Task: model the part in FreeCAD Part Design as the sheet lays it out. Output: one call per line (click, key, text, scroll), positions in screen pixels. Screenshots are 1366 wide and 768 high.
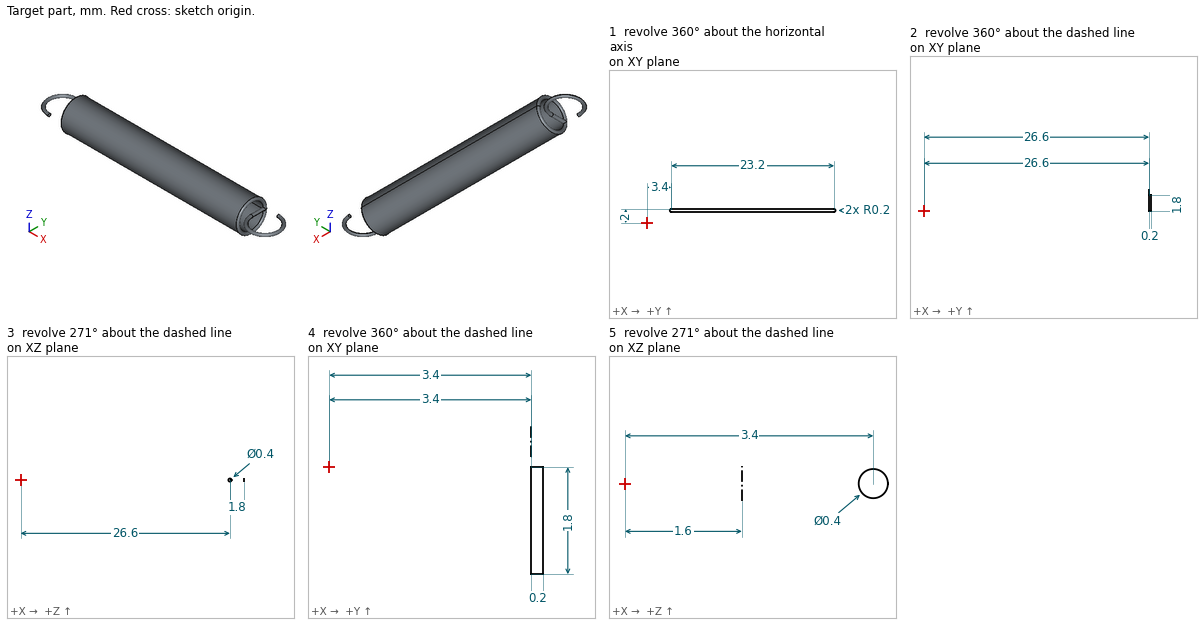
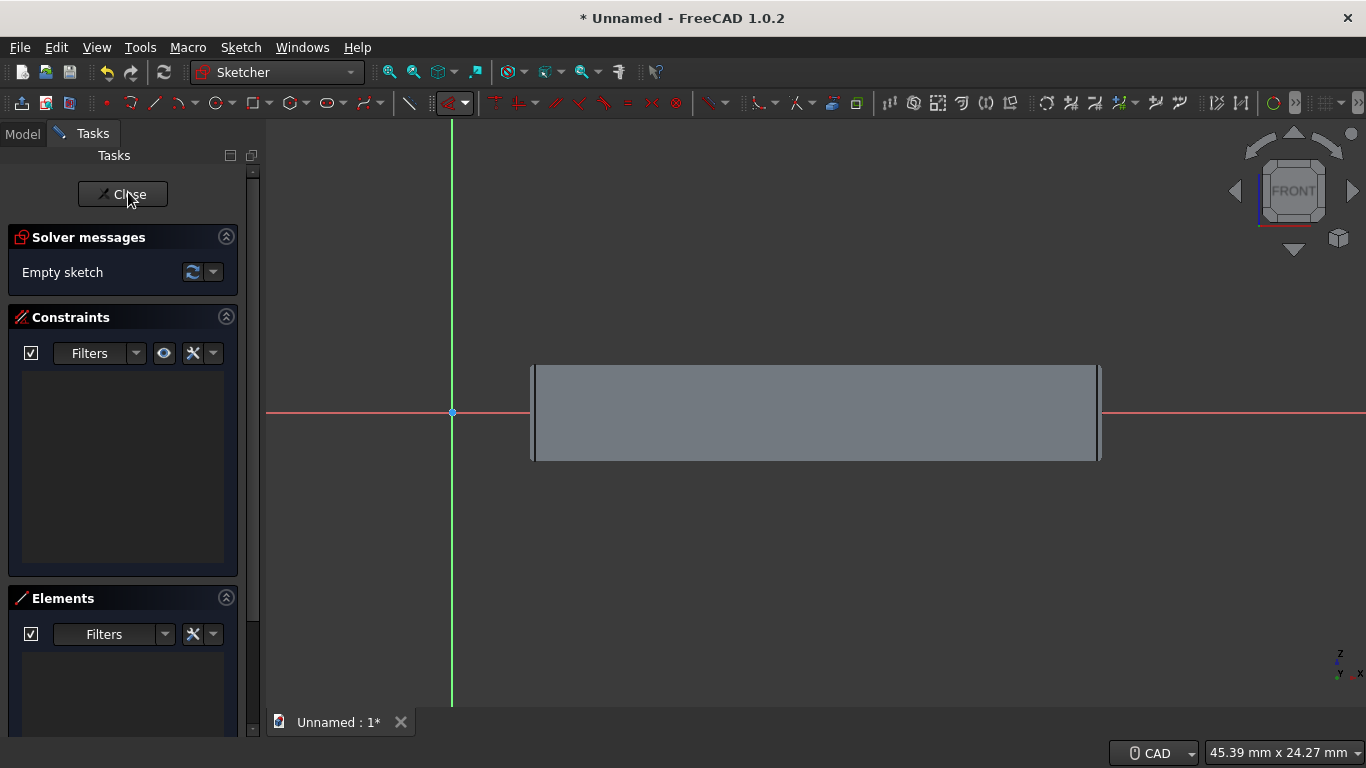
click(70, 104)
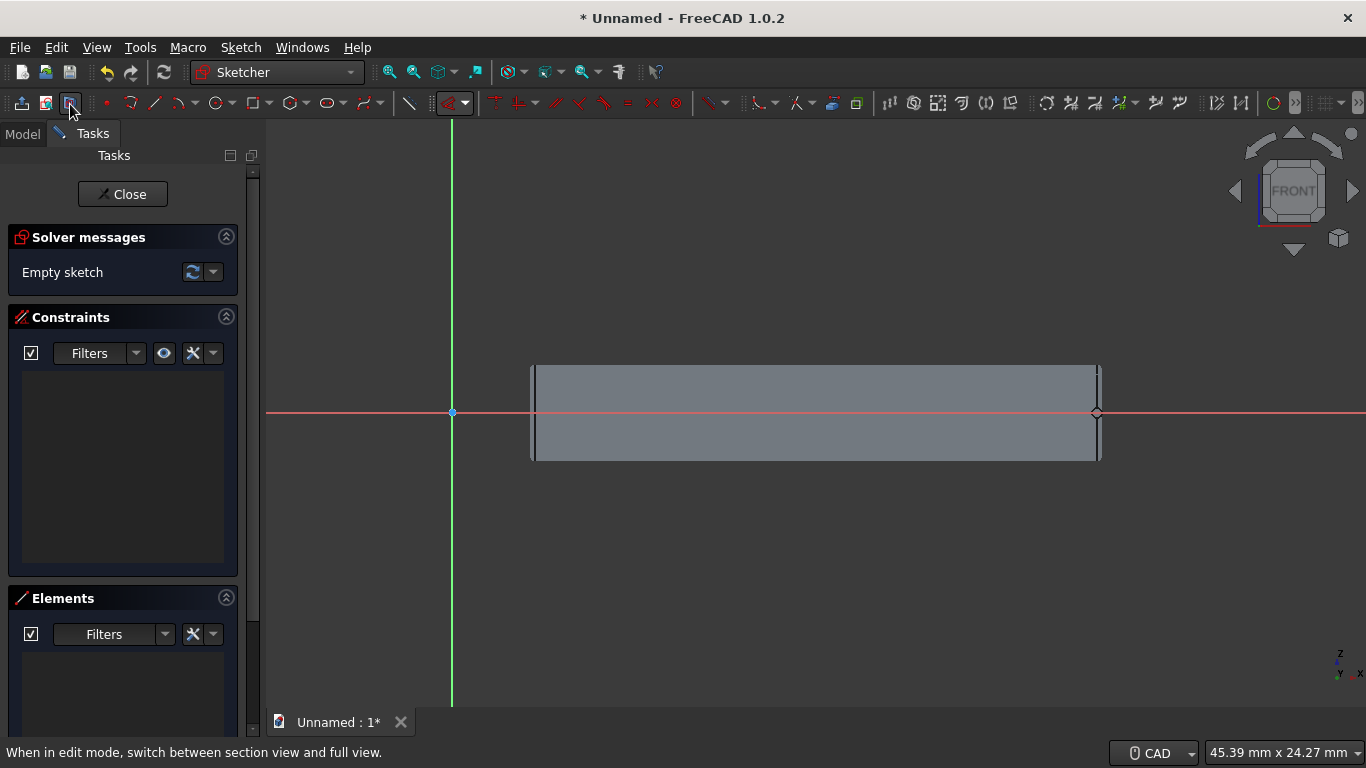
scroll(1146, 413, up, 13)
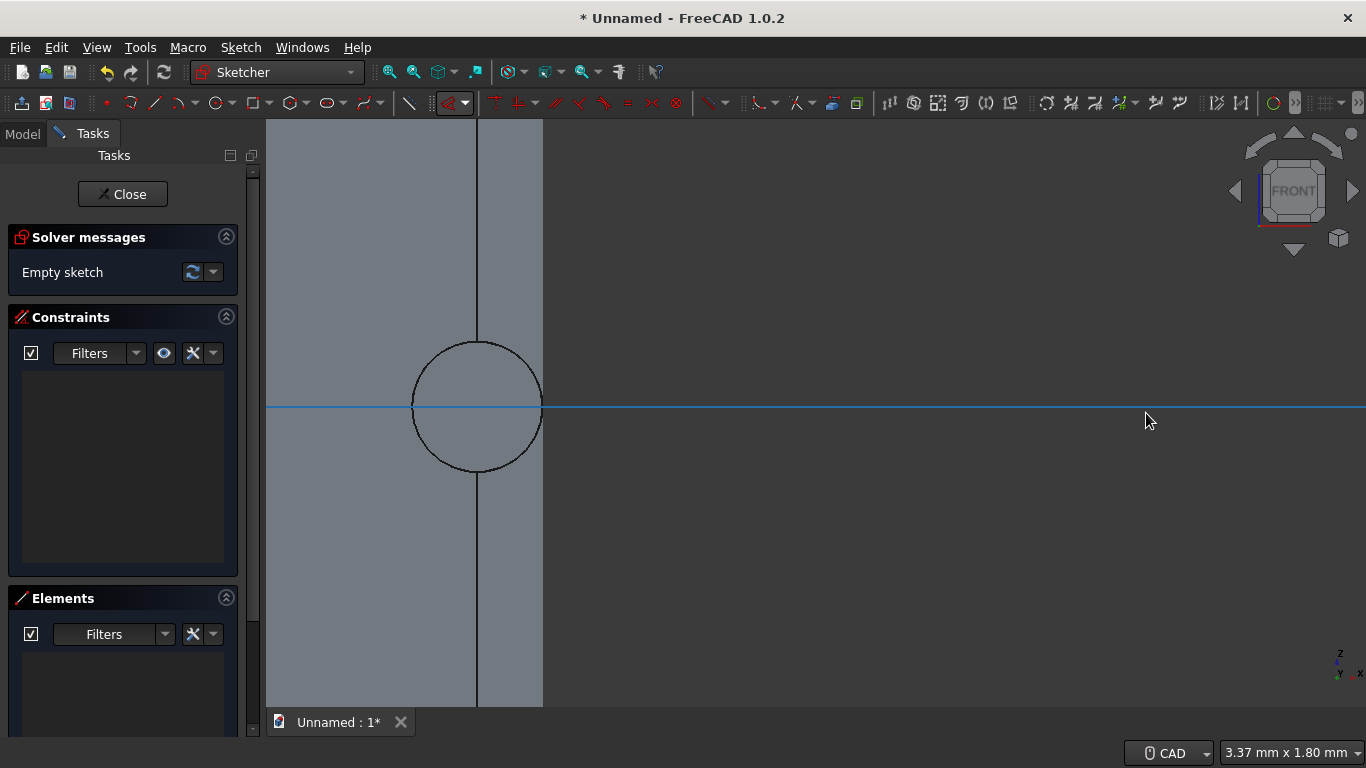
click(216, 104)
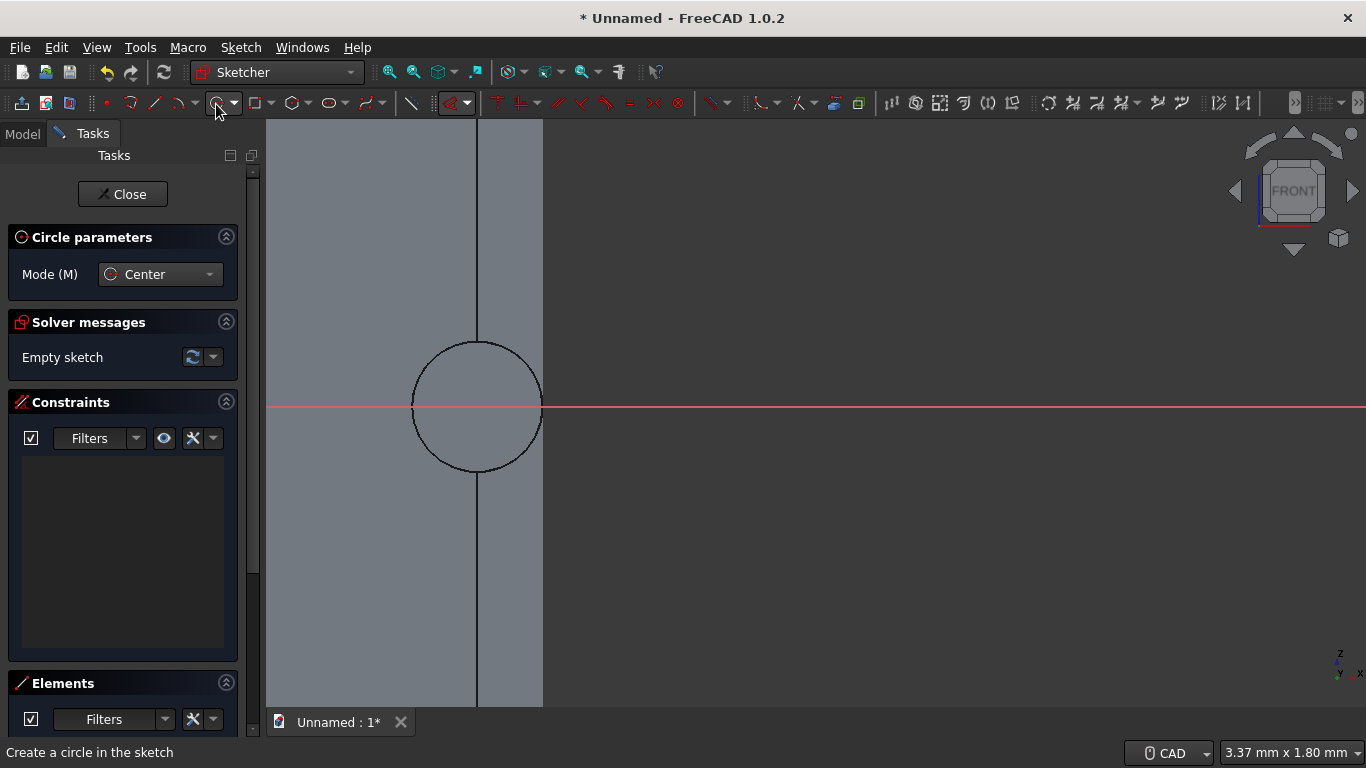
click(477, 407)
click(523, 361)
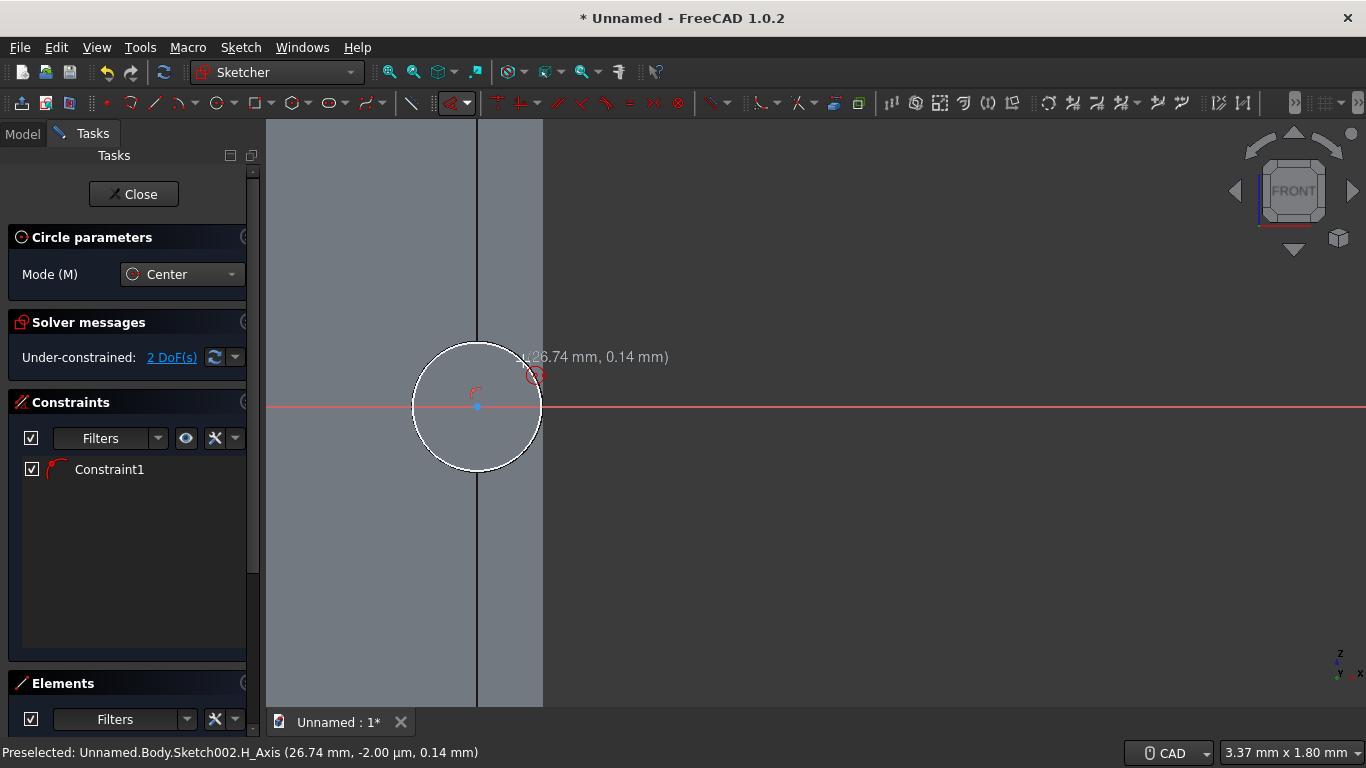
click(156, 104)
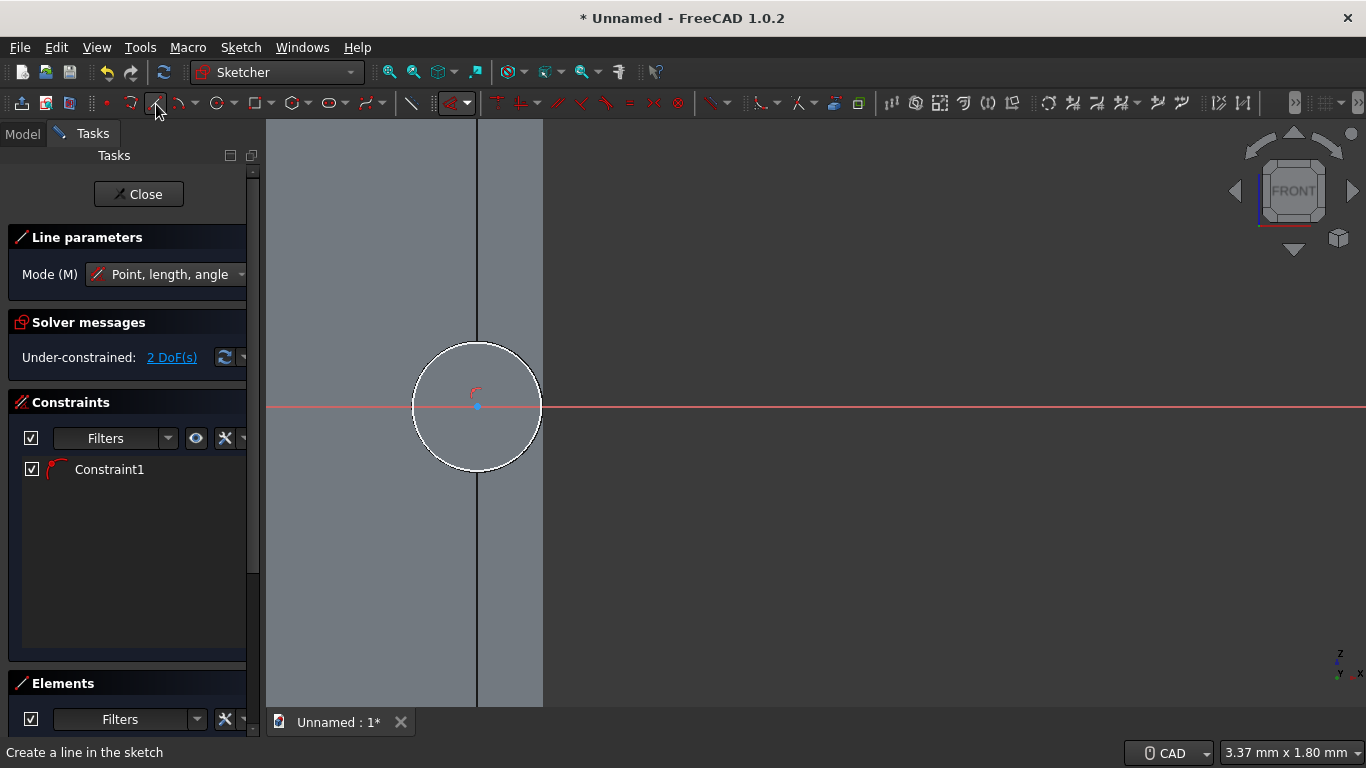
click(1065, 485)
click(1065, 328)
key(Escape)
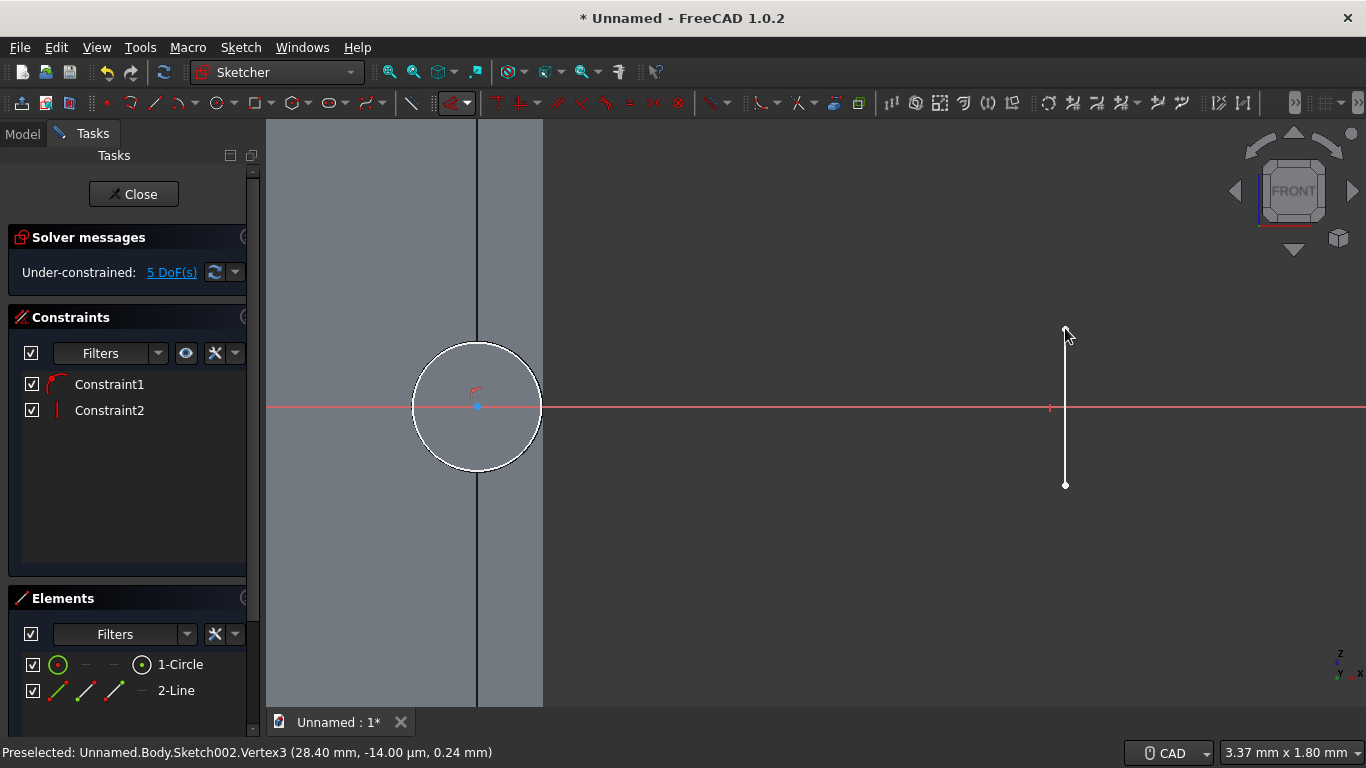
click(1065, 439)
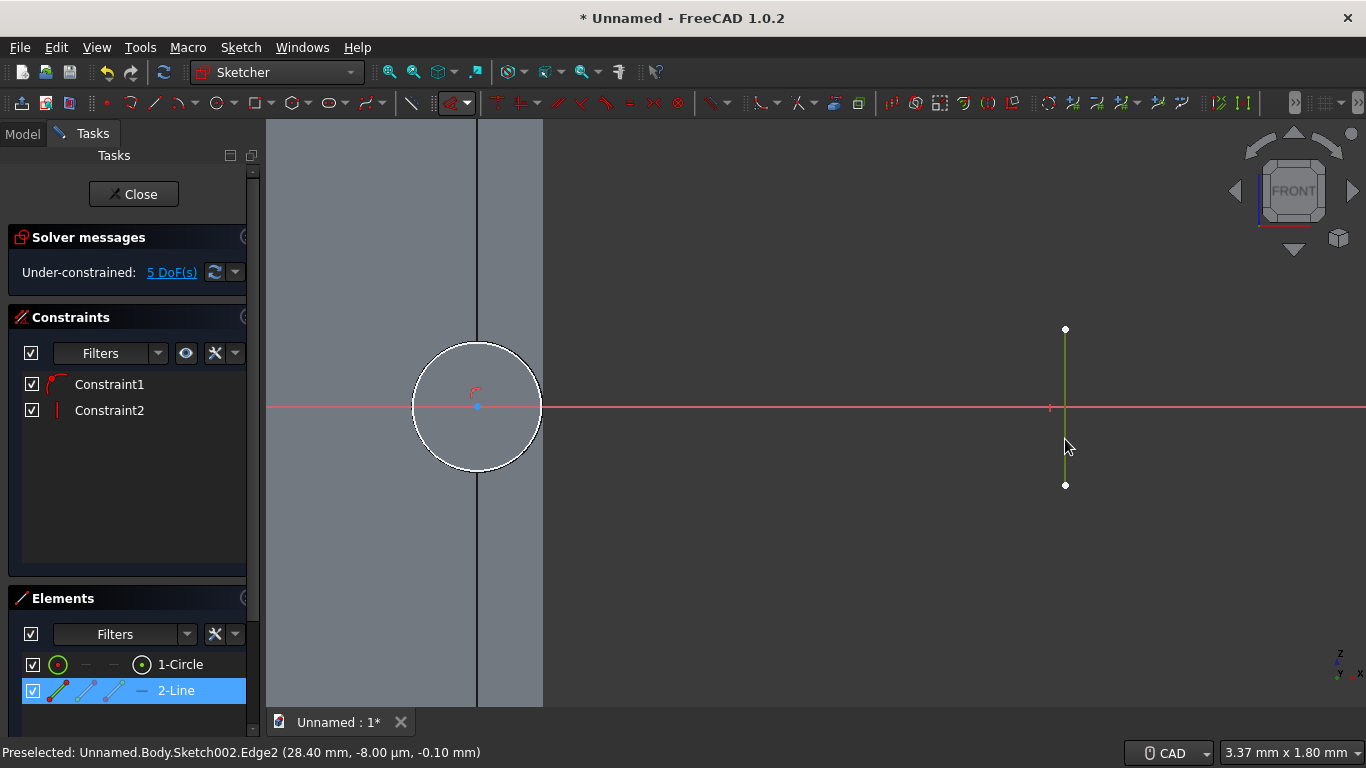
click(412, 104)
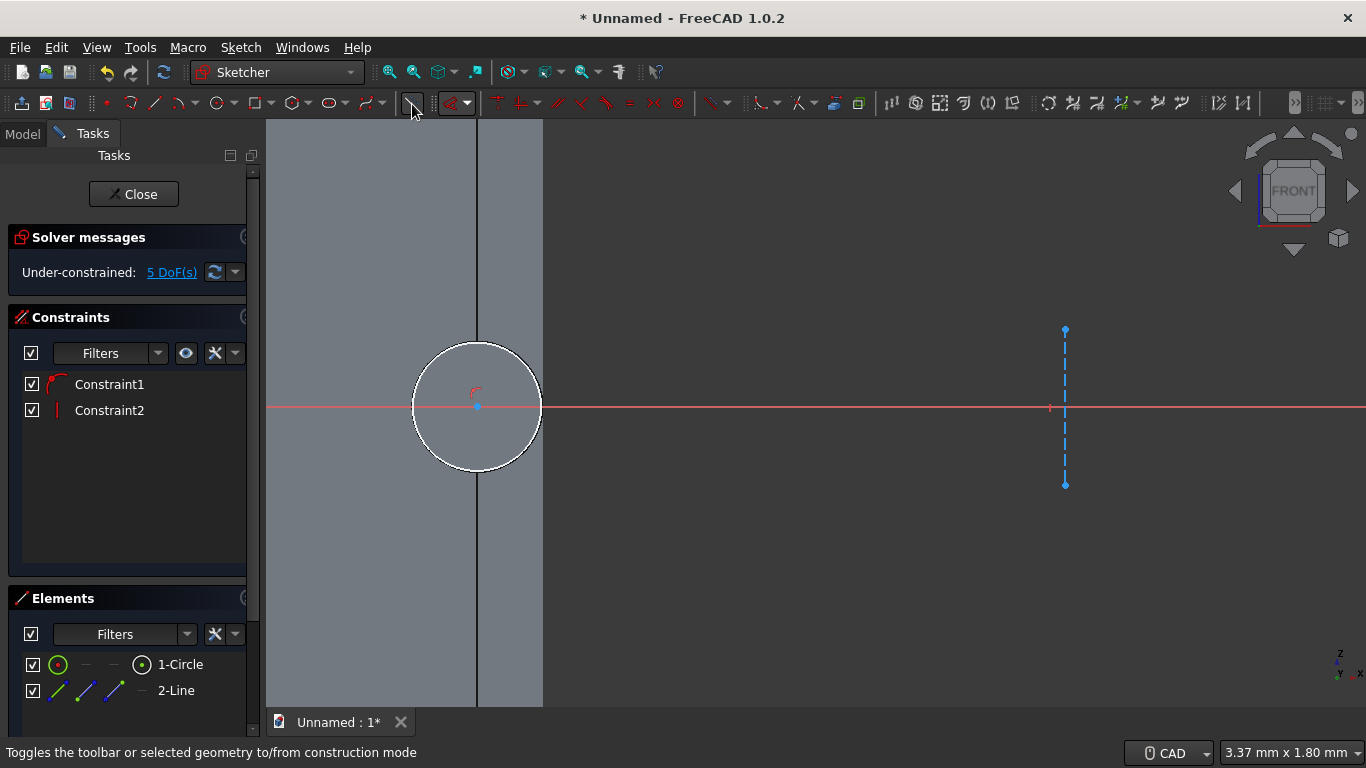
click(522, 361)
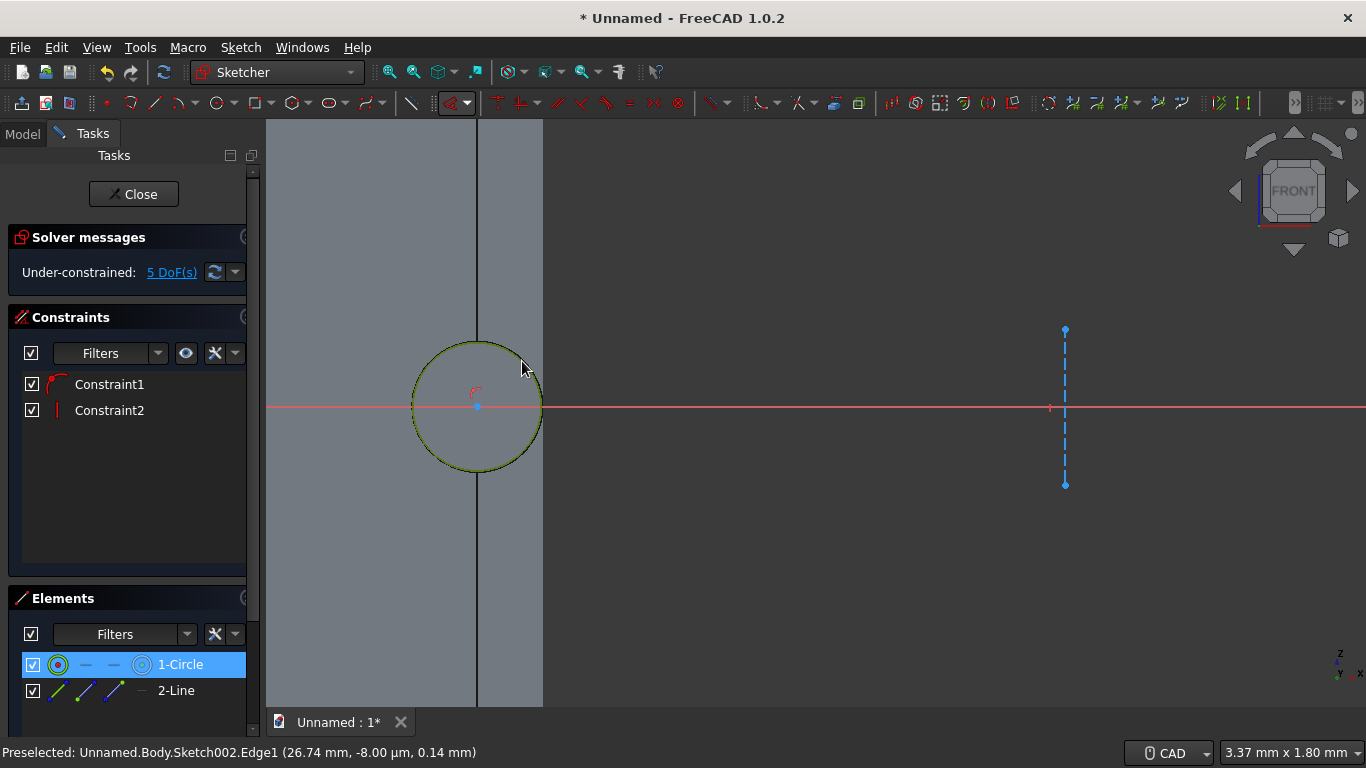
key(k)
key(o)